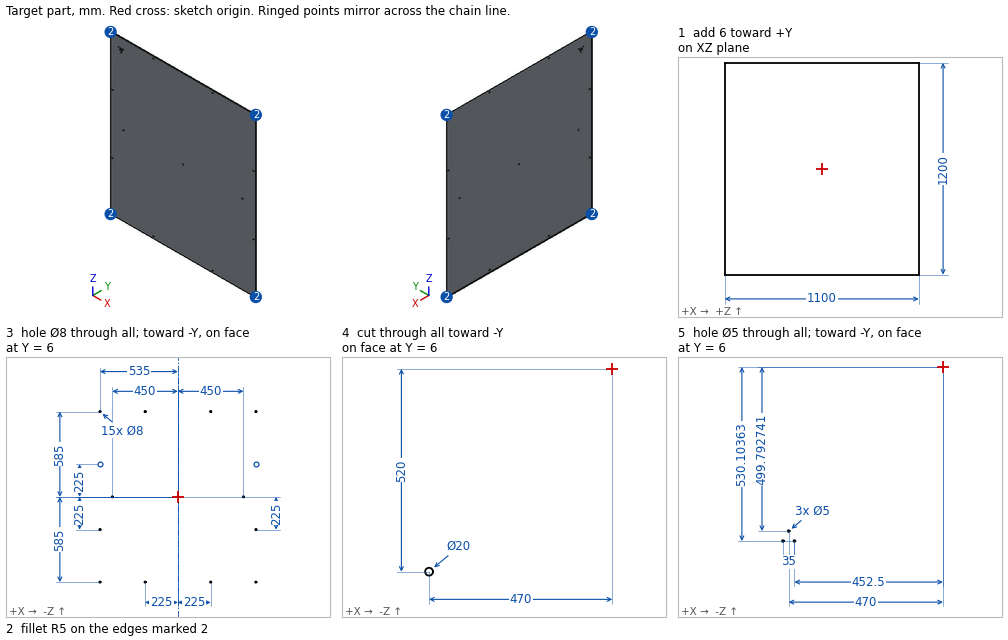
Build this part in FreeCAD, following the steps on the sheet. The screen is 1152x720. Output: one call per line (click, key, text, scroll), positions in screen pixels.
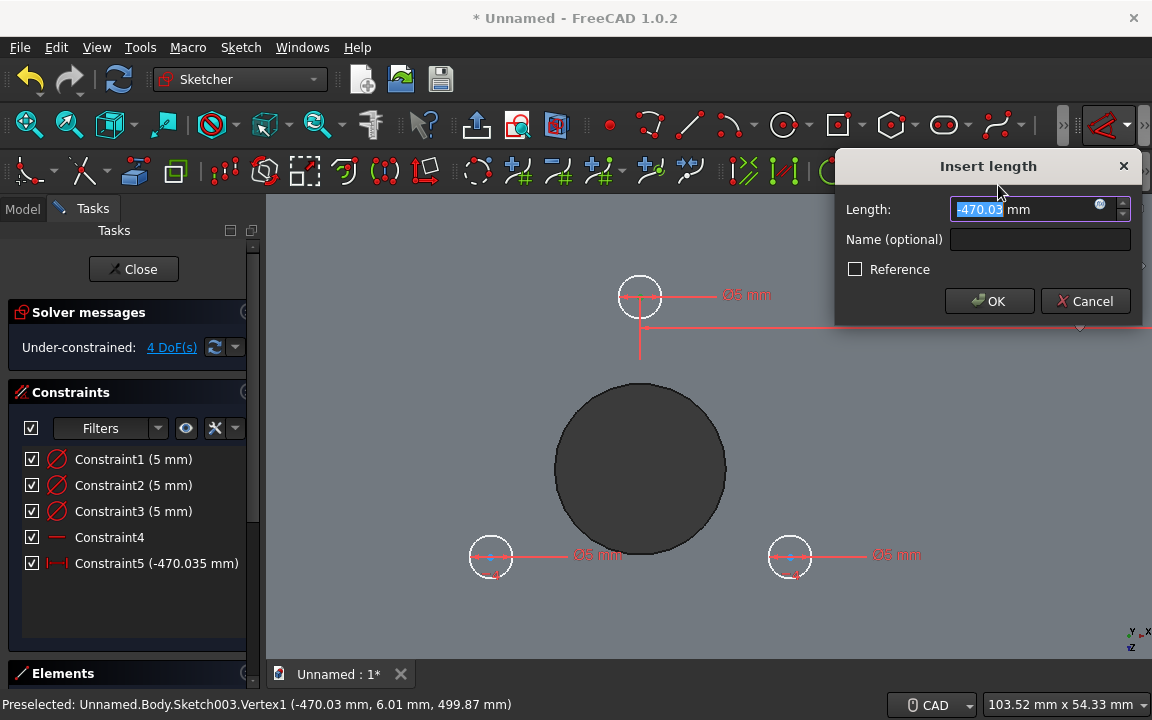
text(-470)
key(Return)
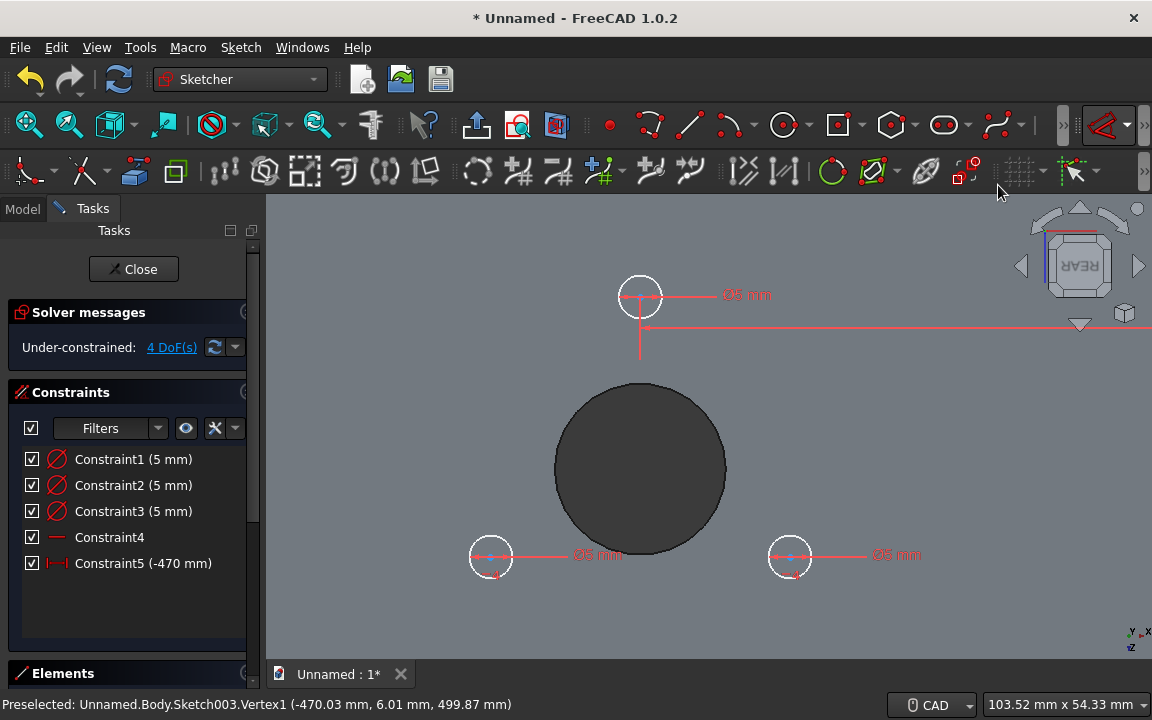
click(790, 557)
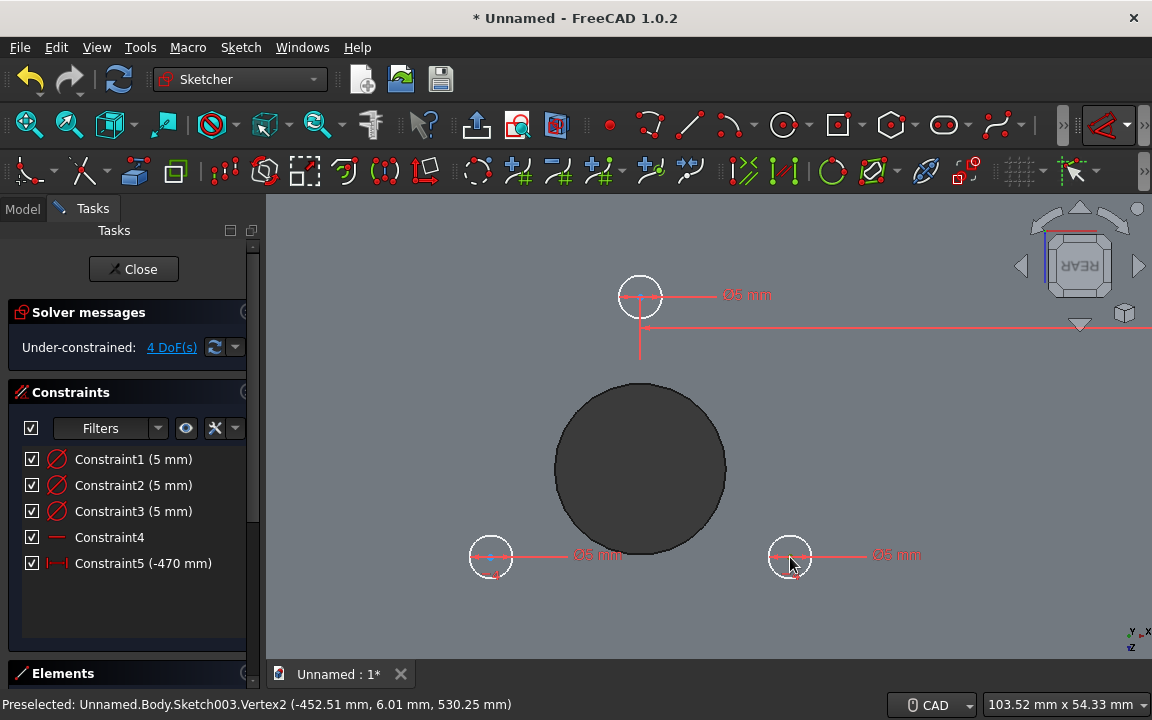
click(491, 557)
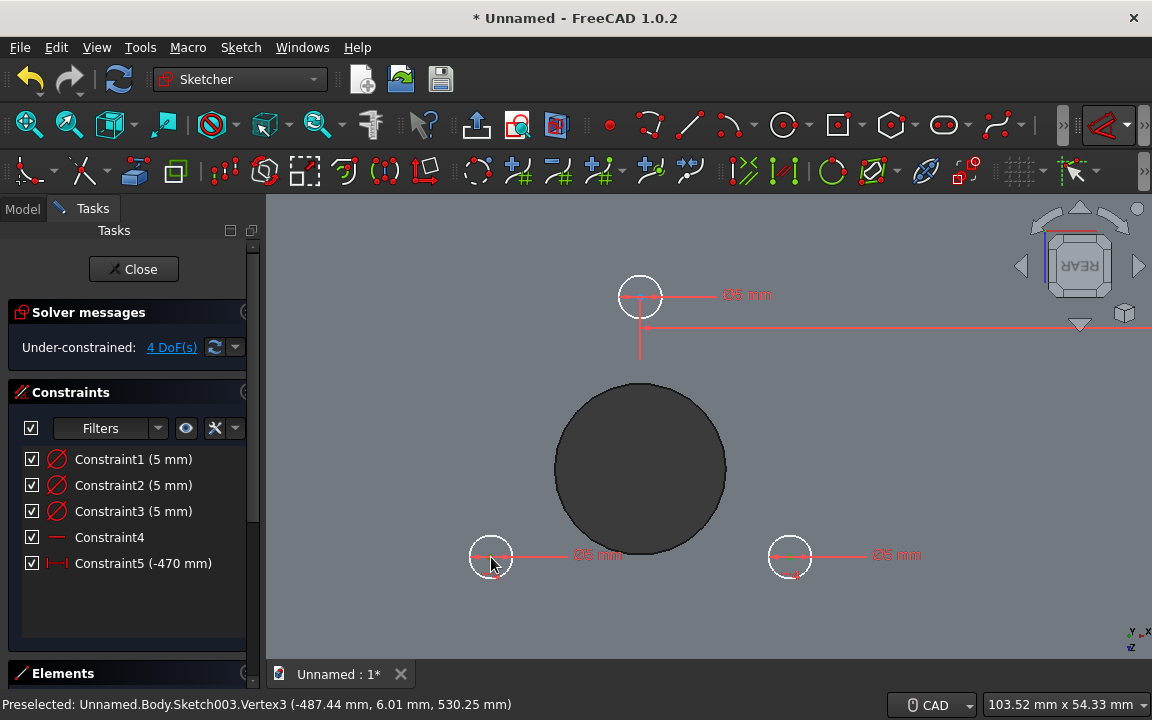
click(1130, 126)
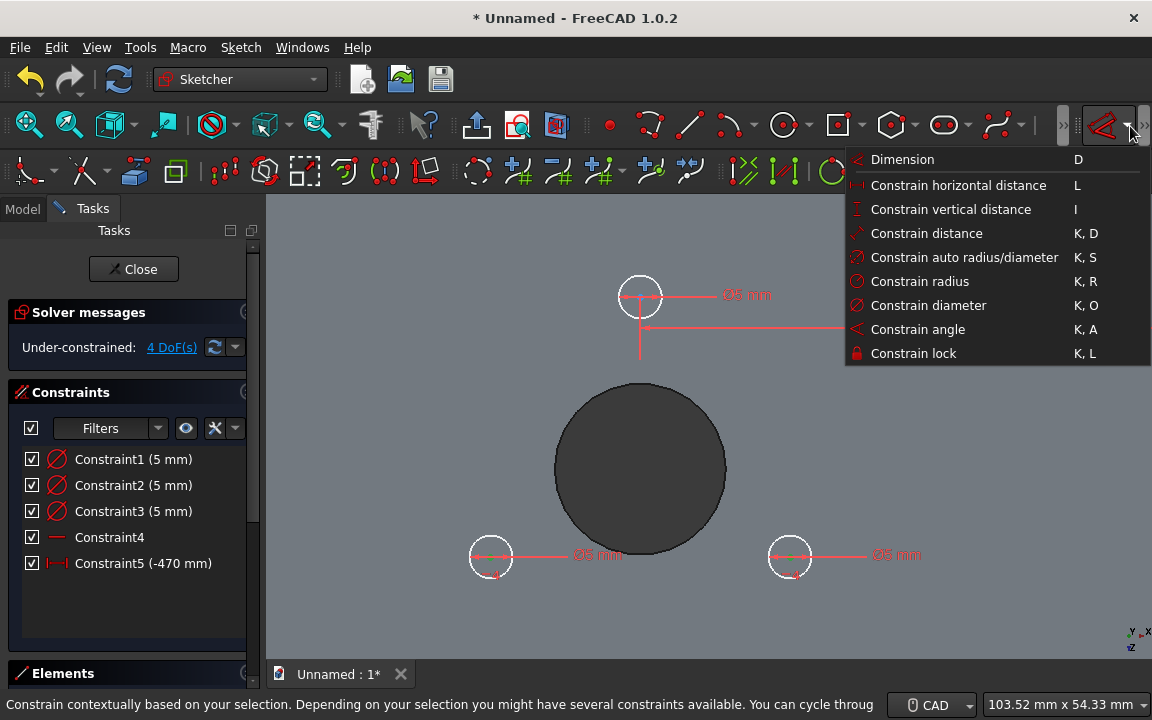
click(998, 185)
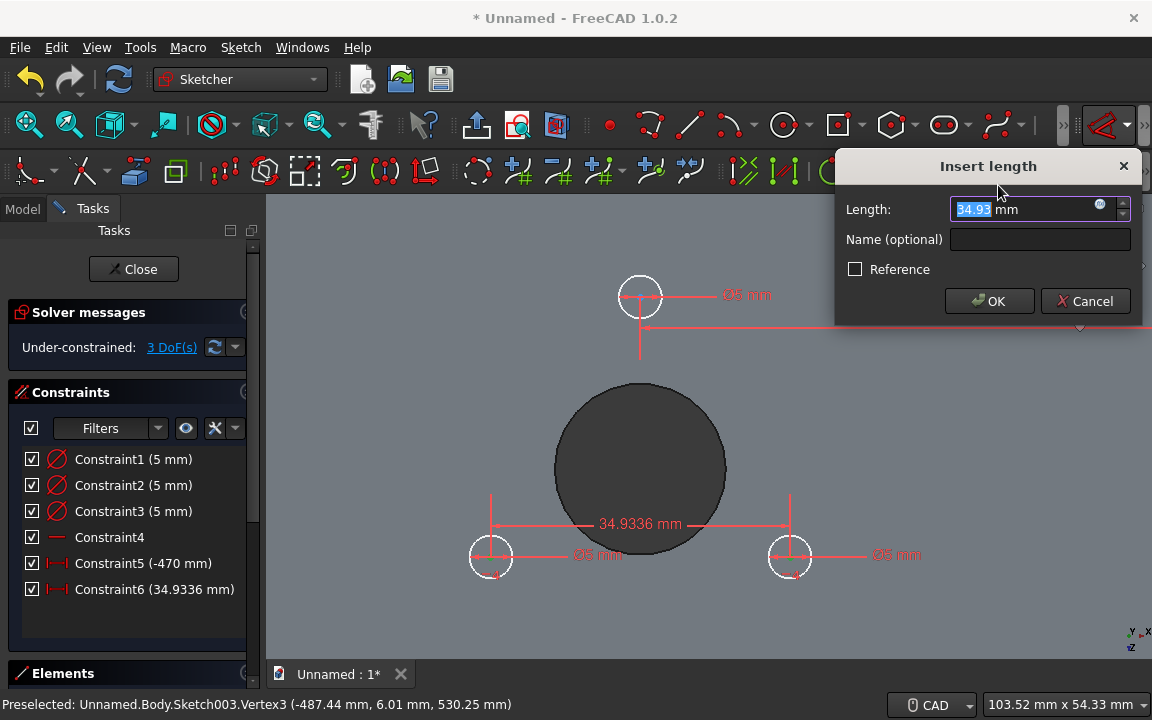
text(35)
key(Return)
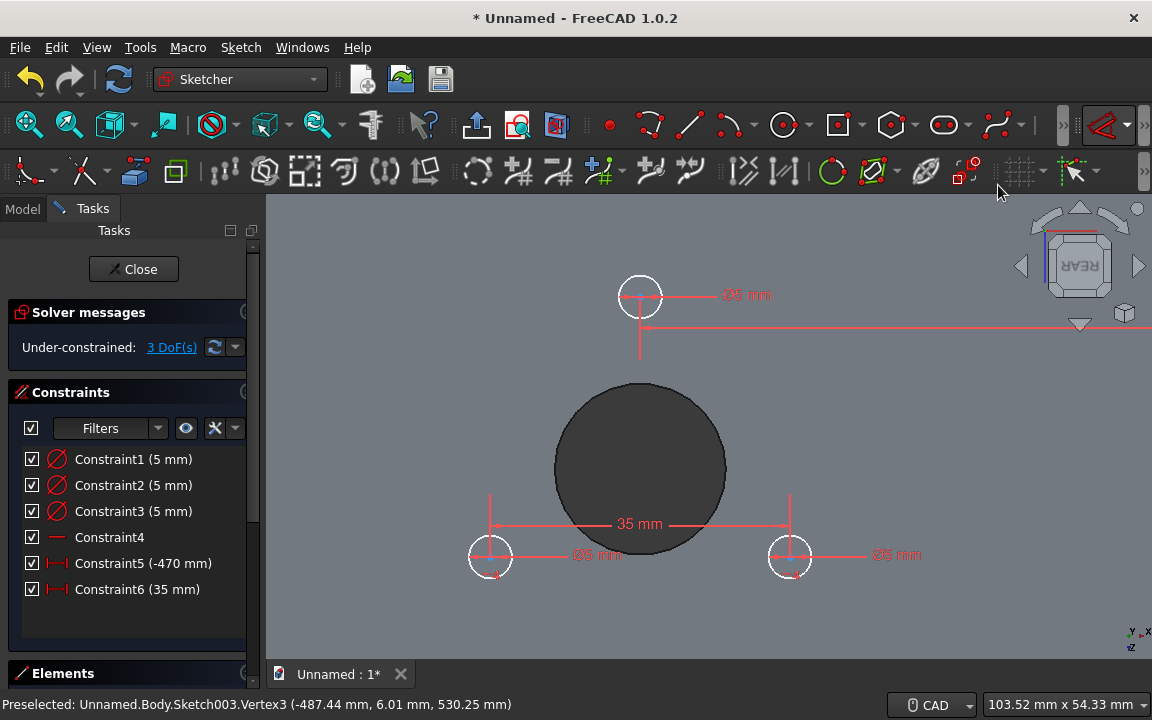
click(790, 557)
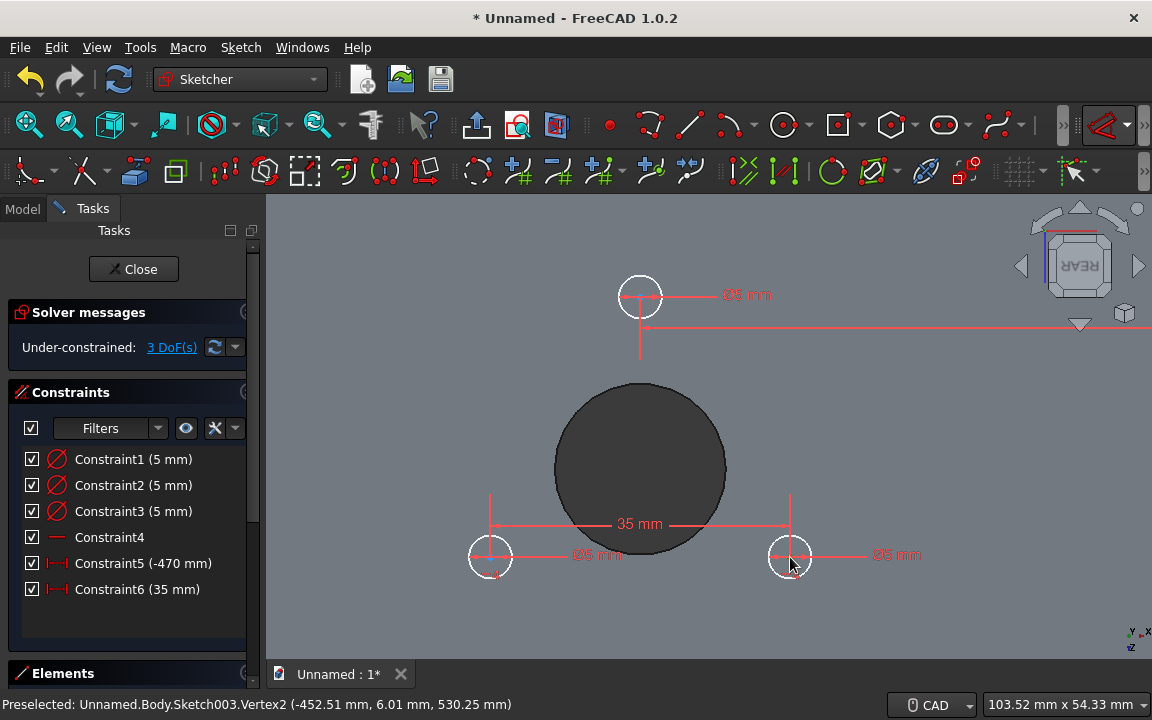
click(1130, 126)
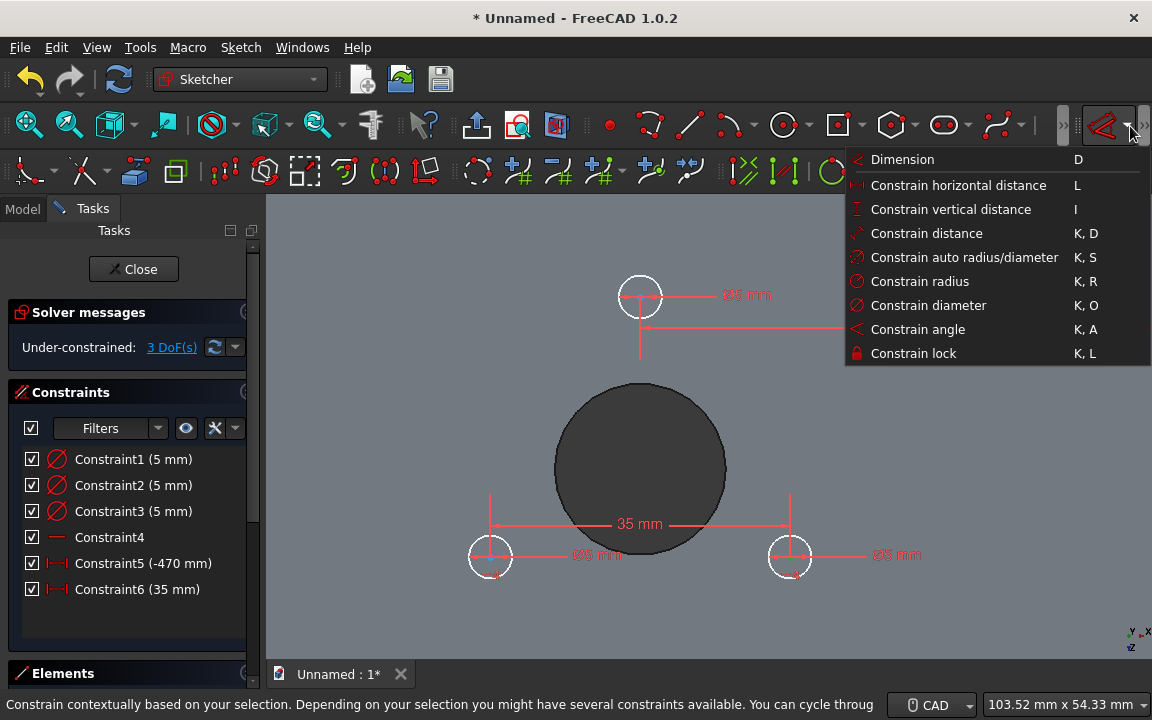
click(998, 185)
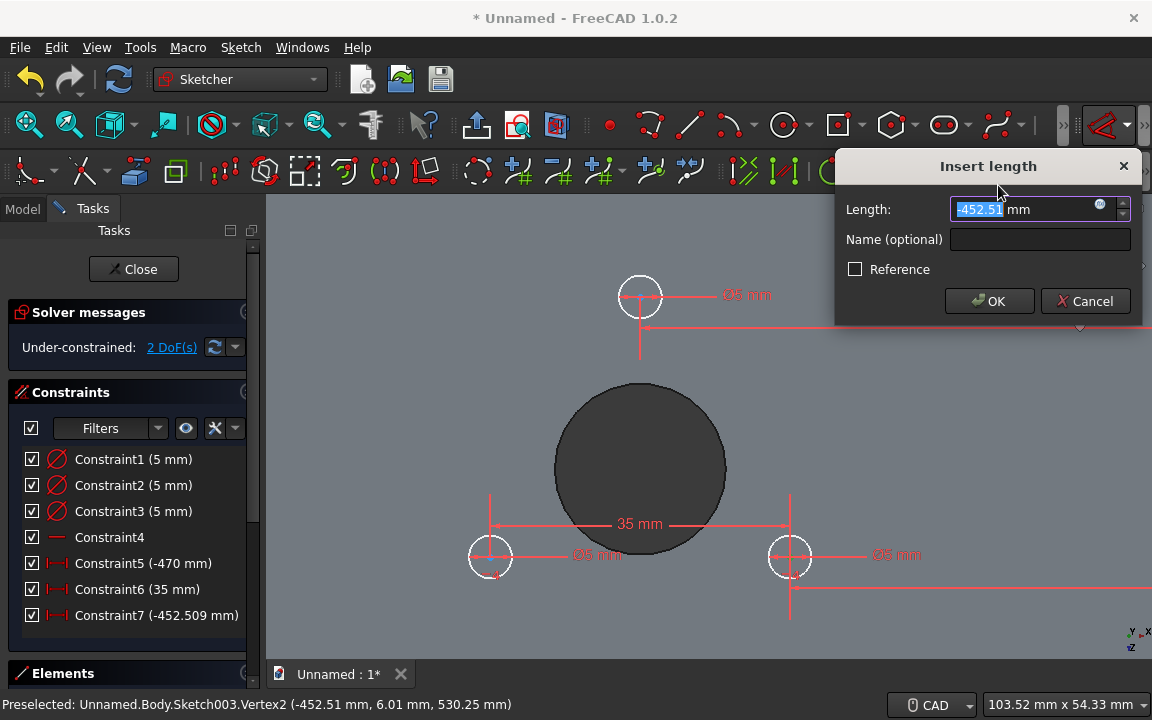
text(-452.5)
key(Return)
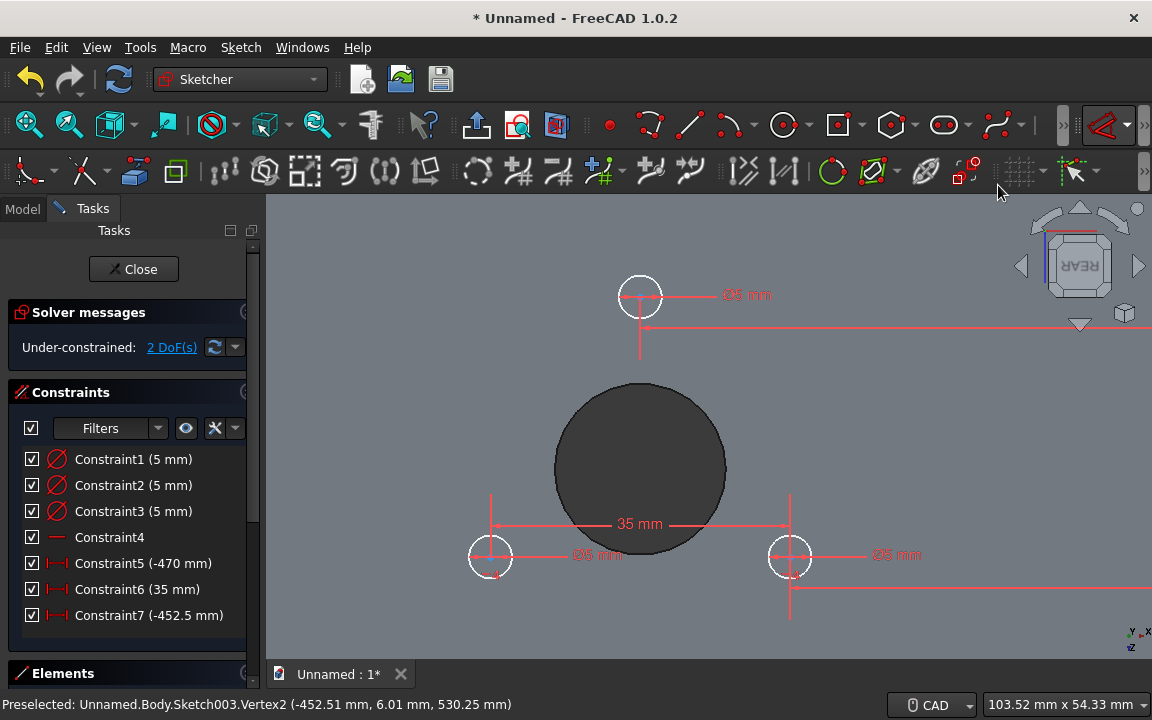
click(790, 557)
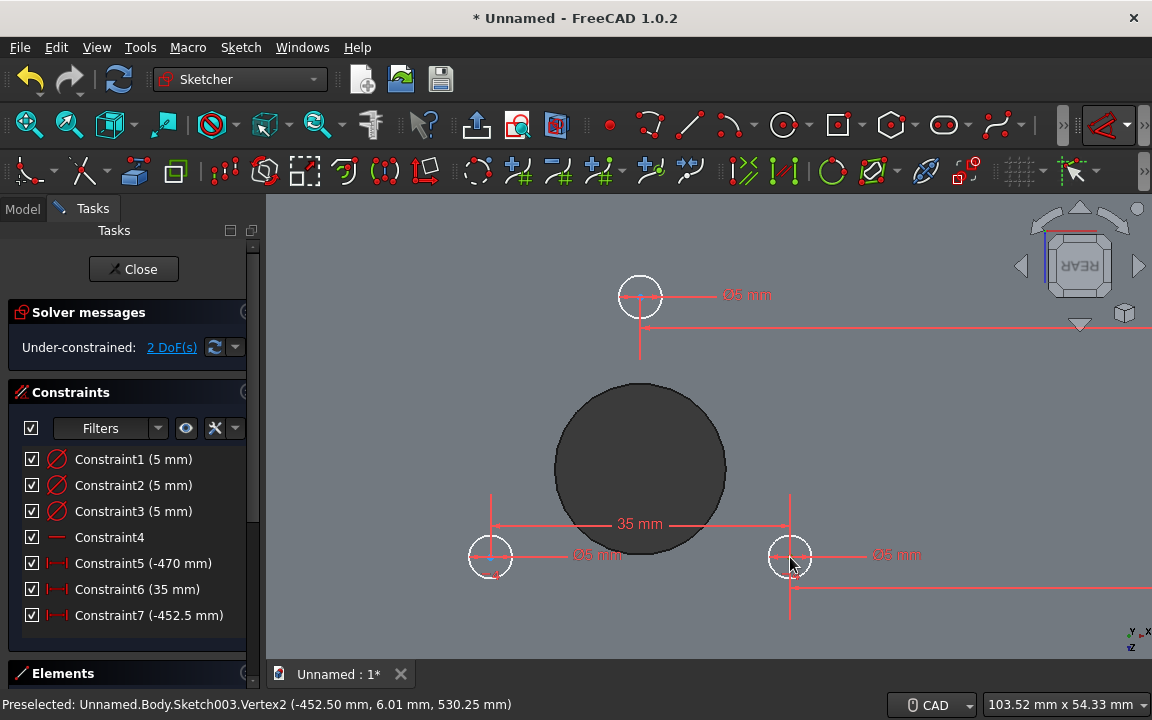
key(i)